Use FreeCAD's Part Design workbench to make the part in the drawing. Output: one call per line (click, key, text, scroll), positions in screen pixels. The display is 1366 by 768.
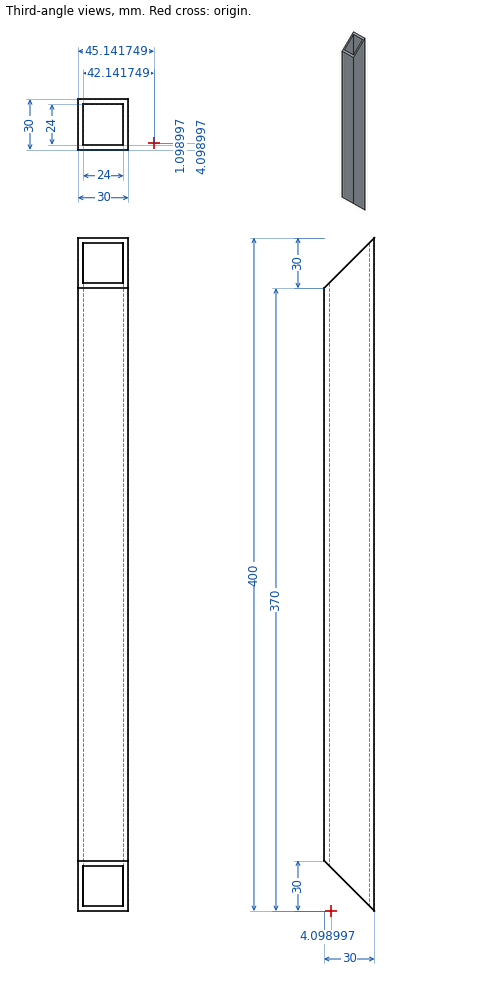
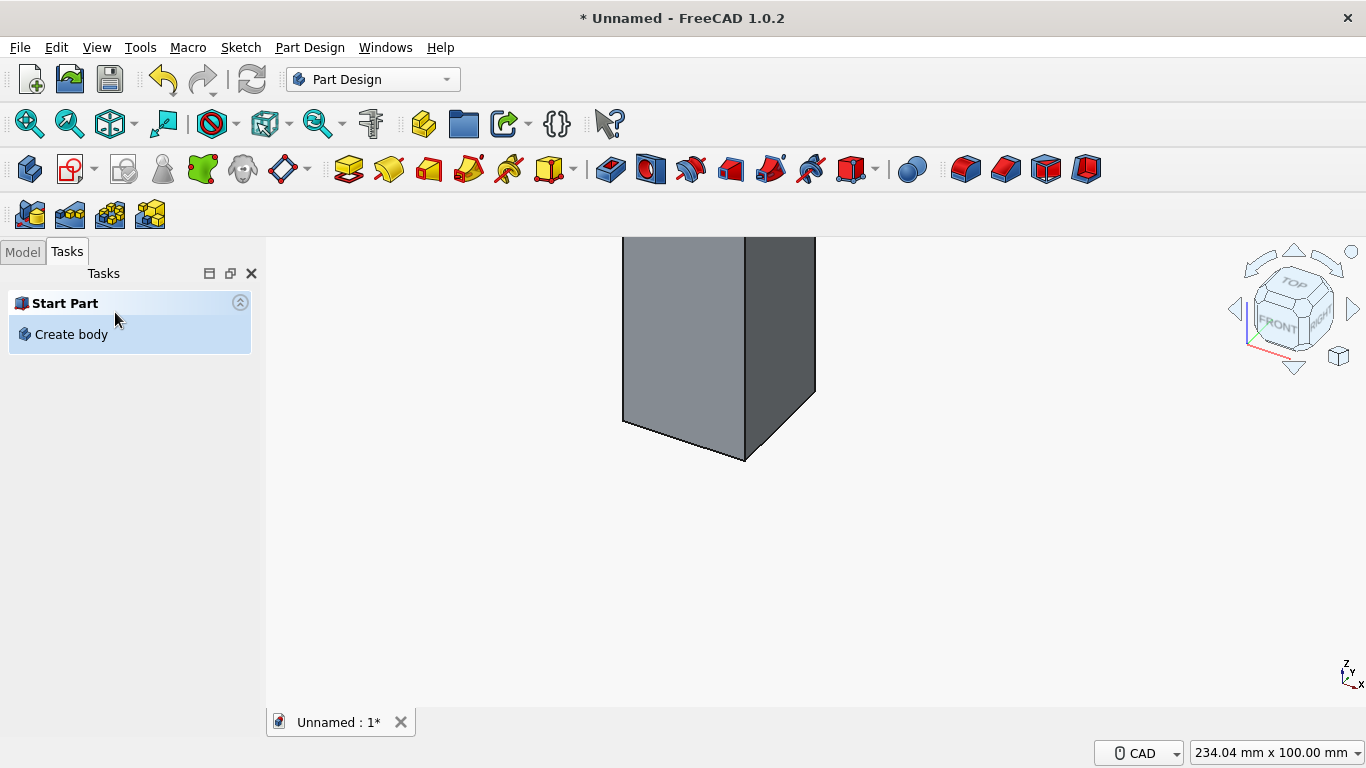
click(30, 124)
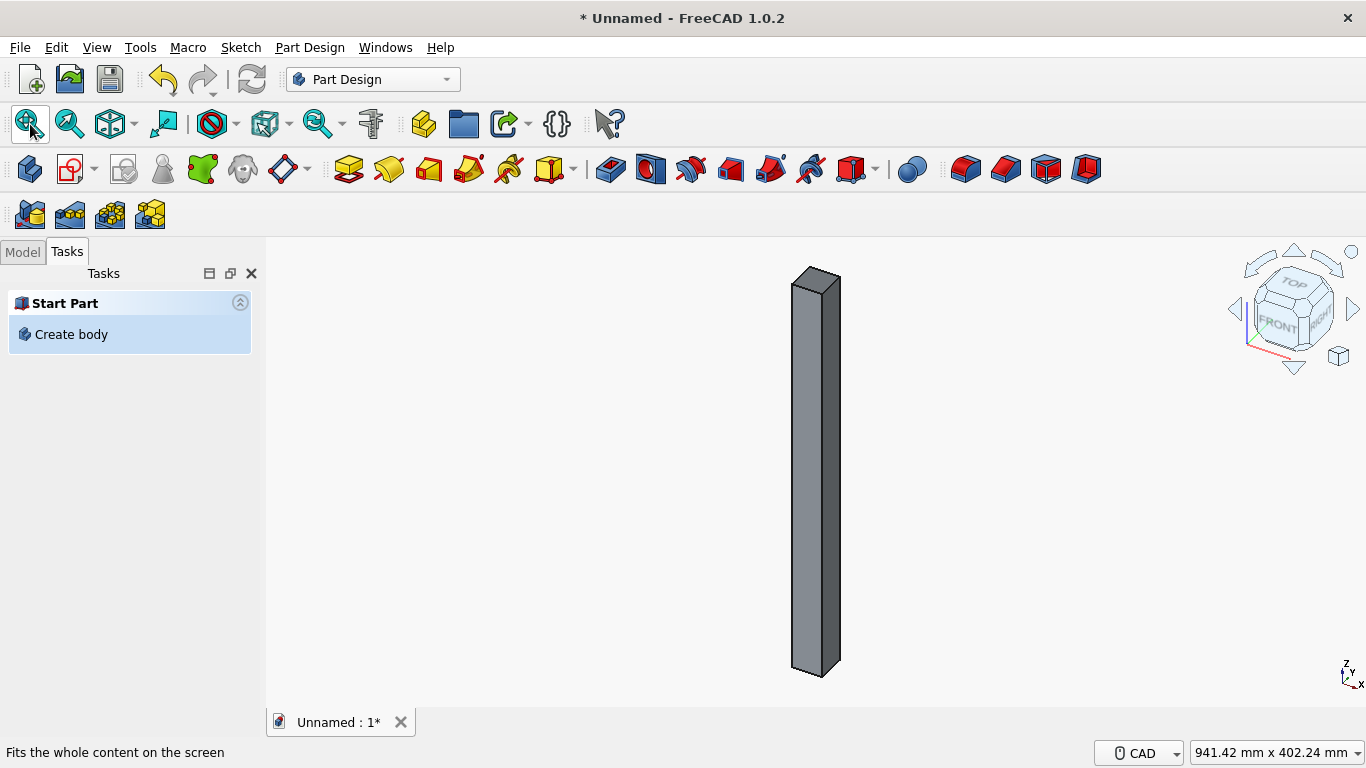
click(816, 280)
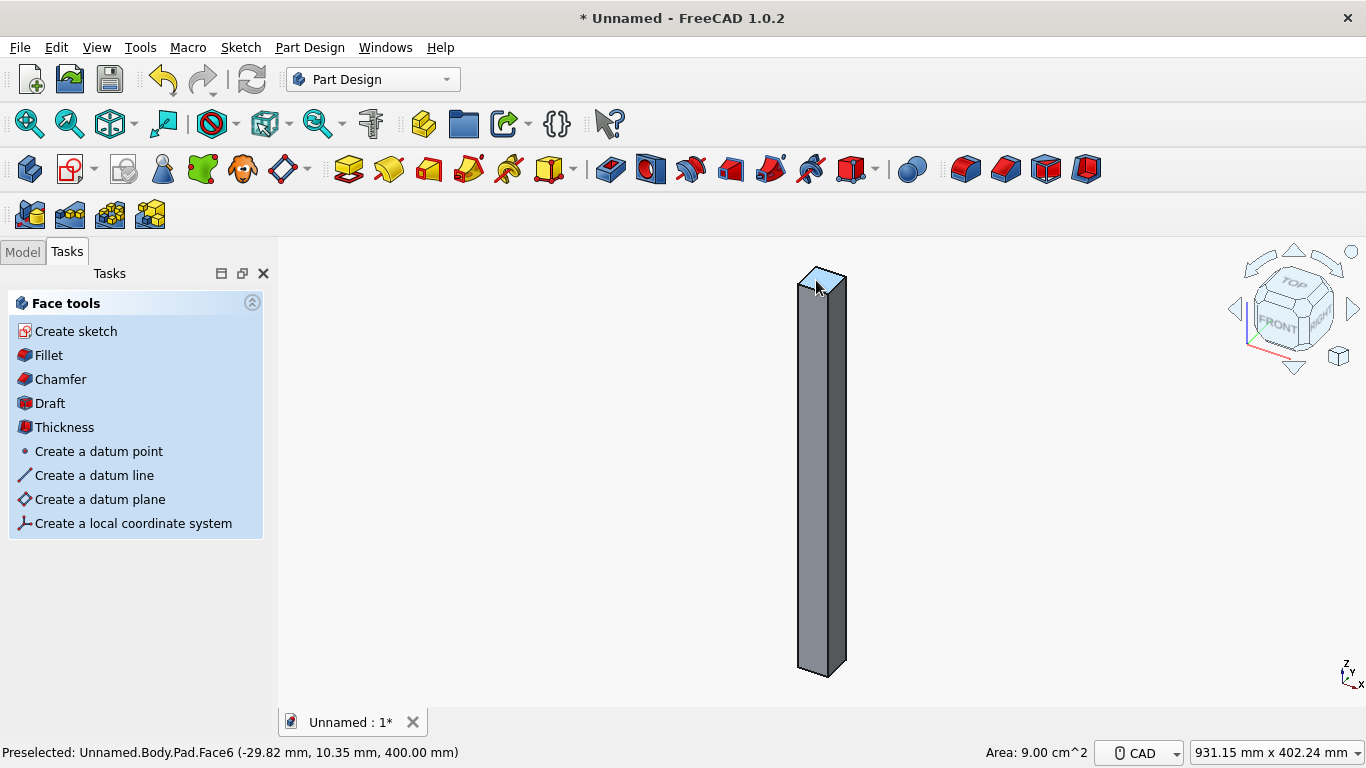
click(70, 170)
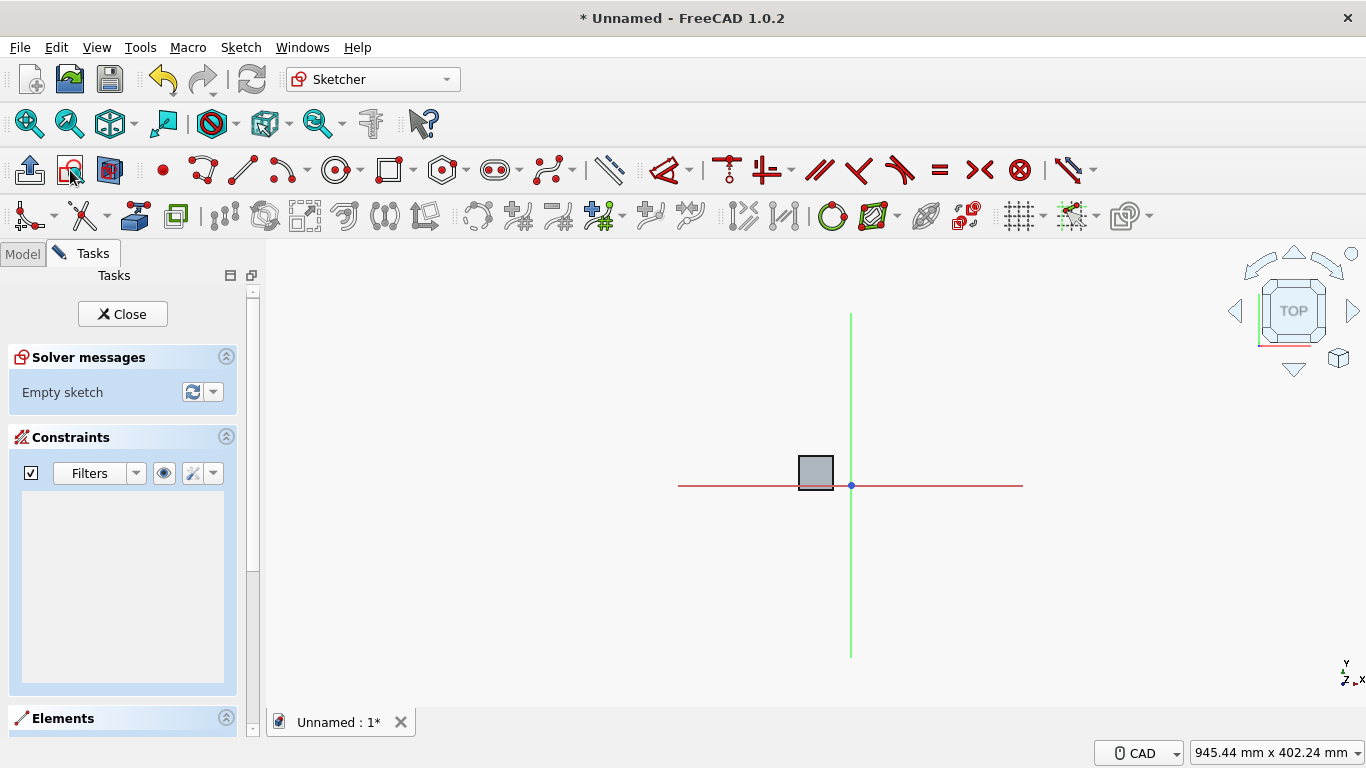
scroll(834, 473, up, 12)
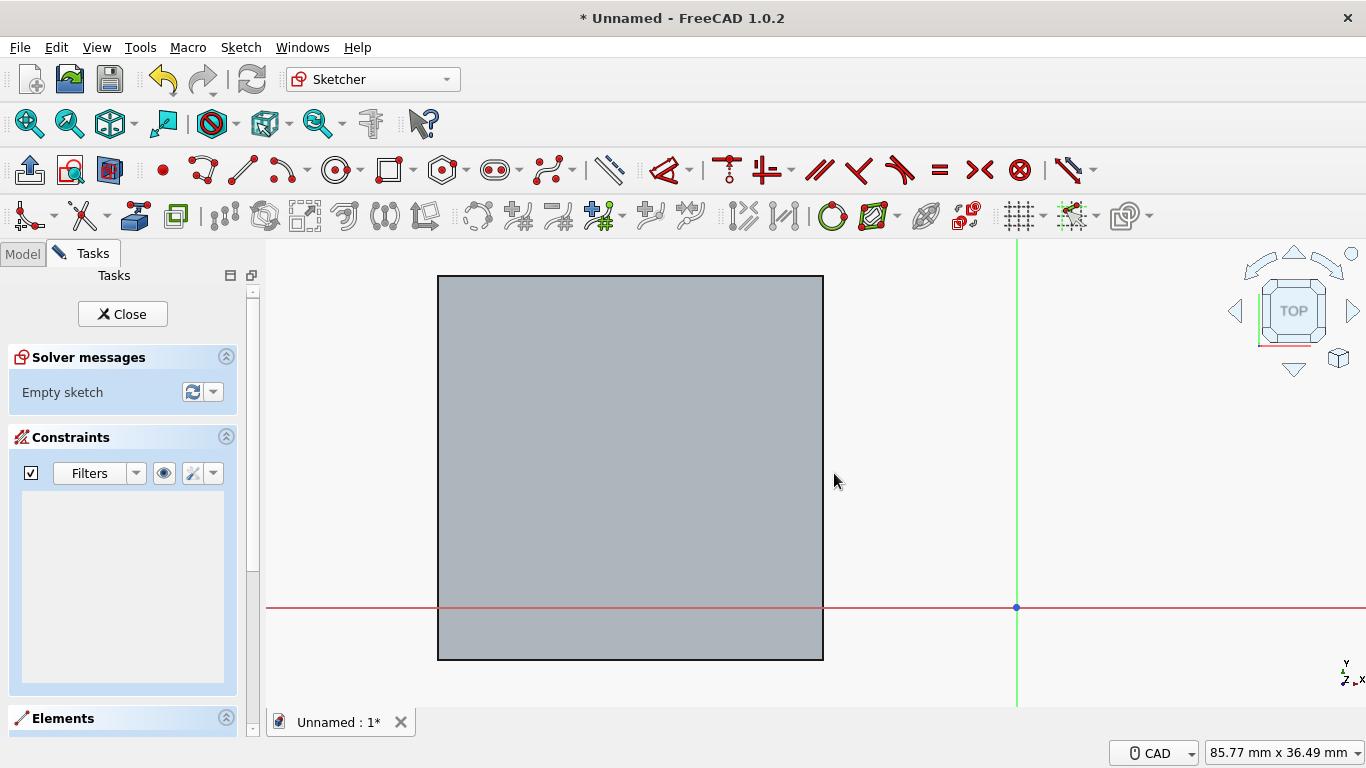
click(390, 170)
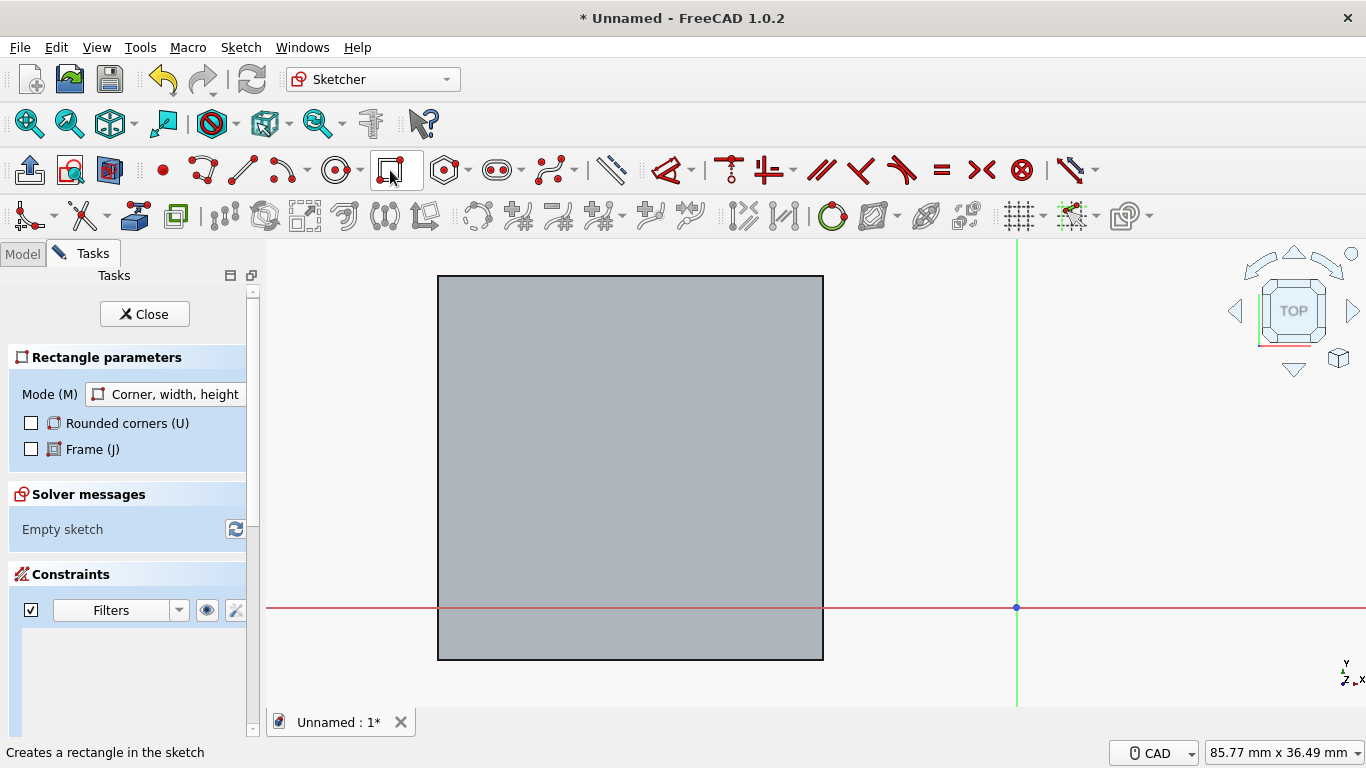
click(477, 314)
click(784, 622)
key(Escape)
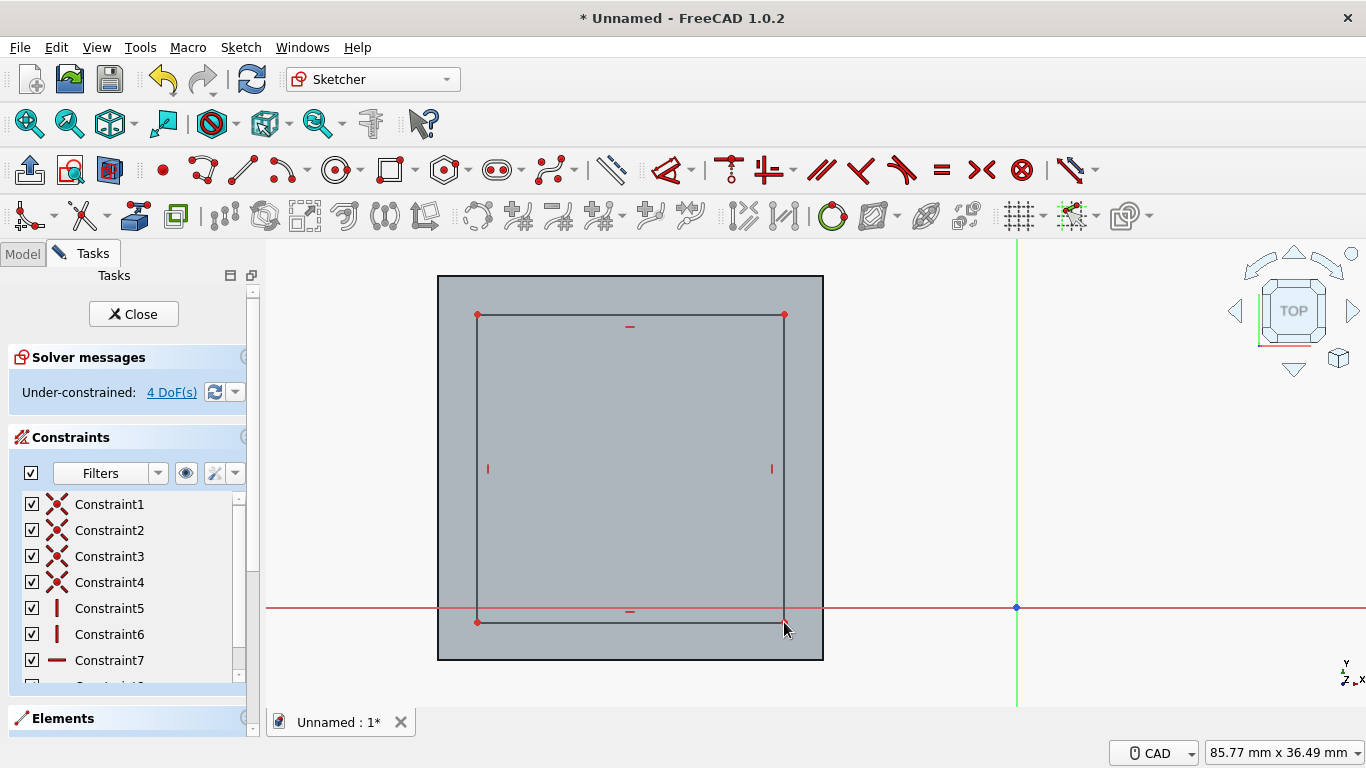
key(d)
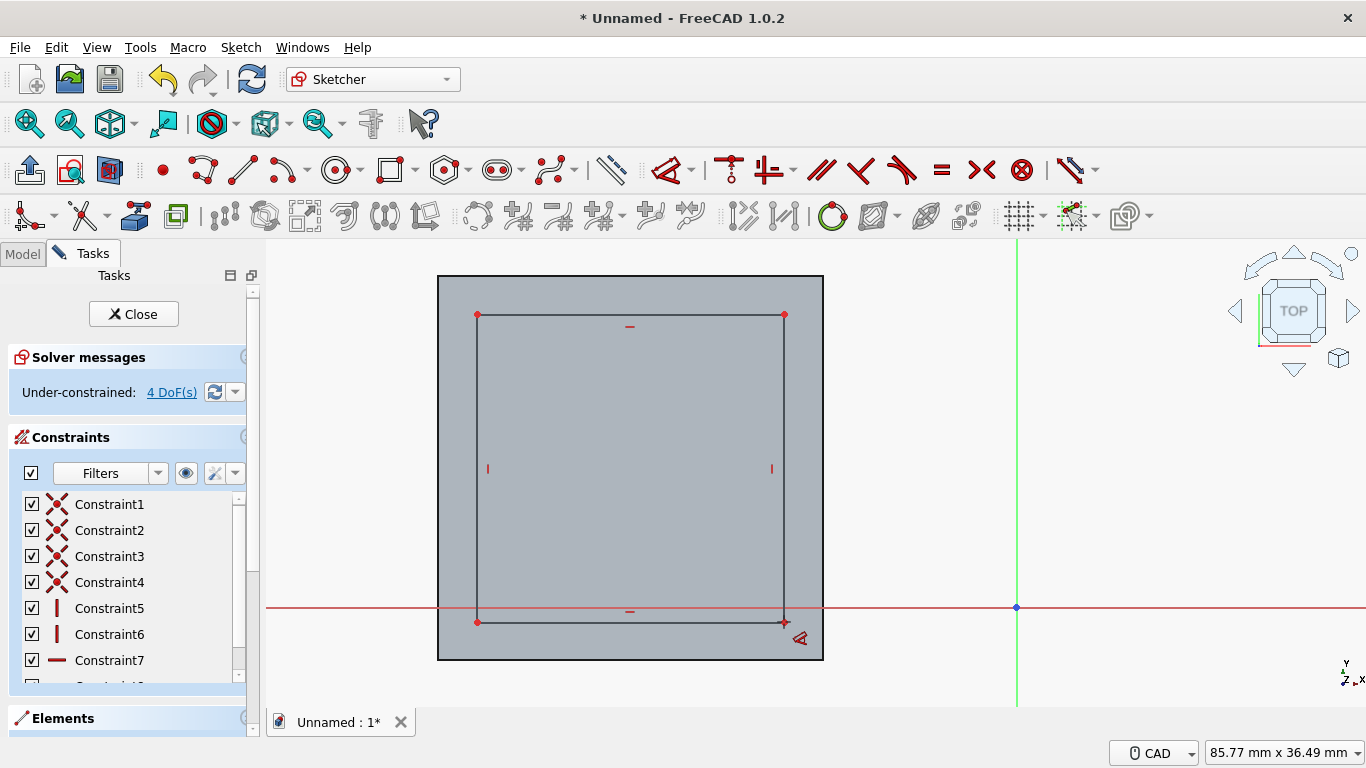
click(477, 407)
click(443, 469)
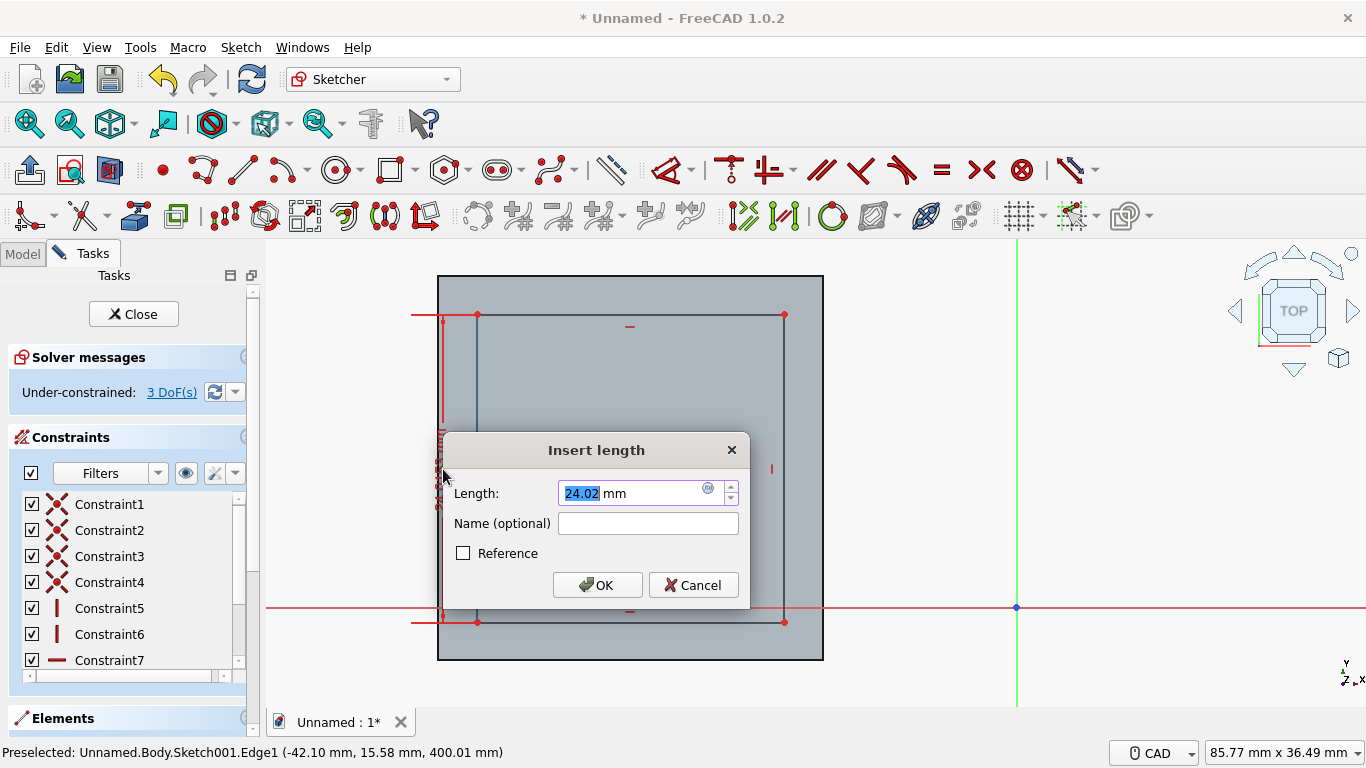
text(24)
key(Return)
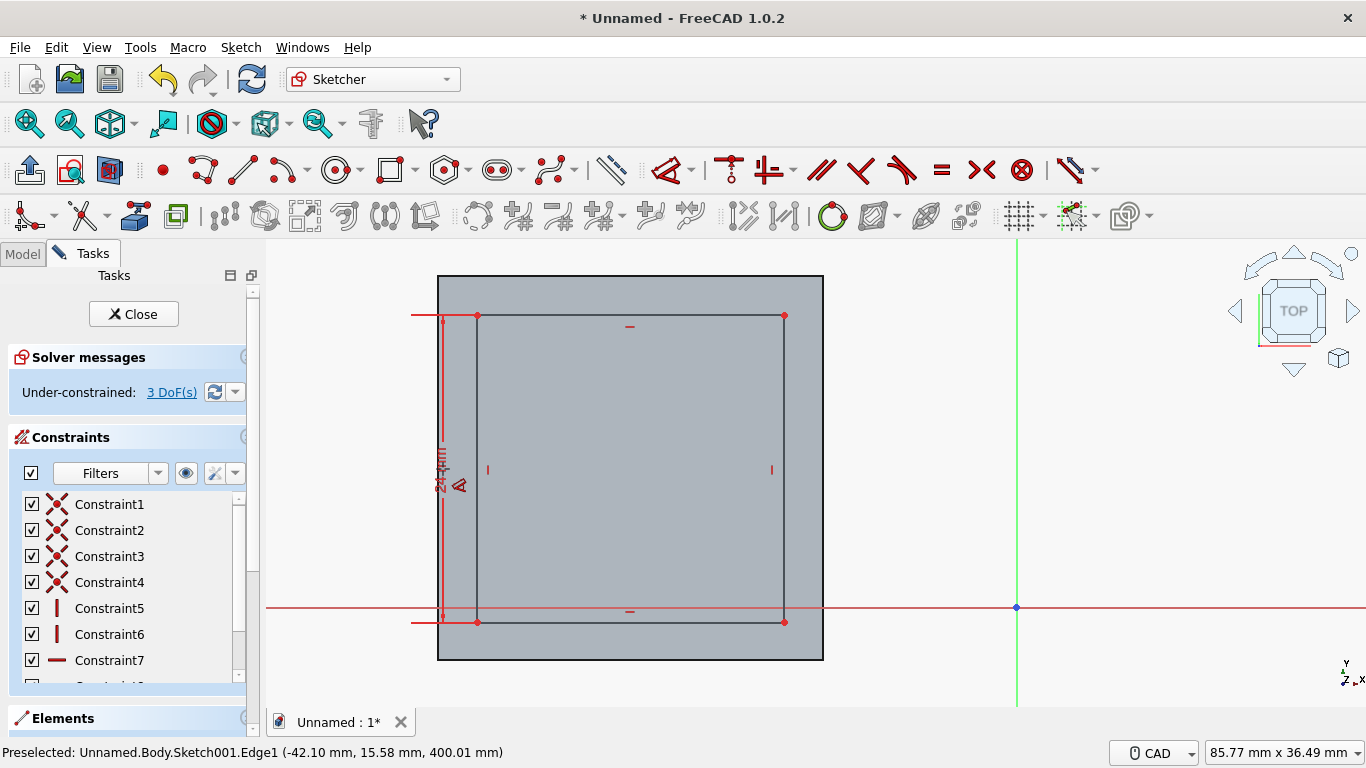
click(569, 623)
click(631, 657)